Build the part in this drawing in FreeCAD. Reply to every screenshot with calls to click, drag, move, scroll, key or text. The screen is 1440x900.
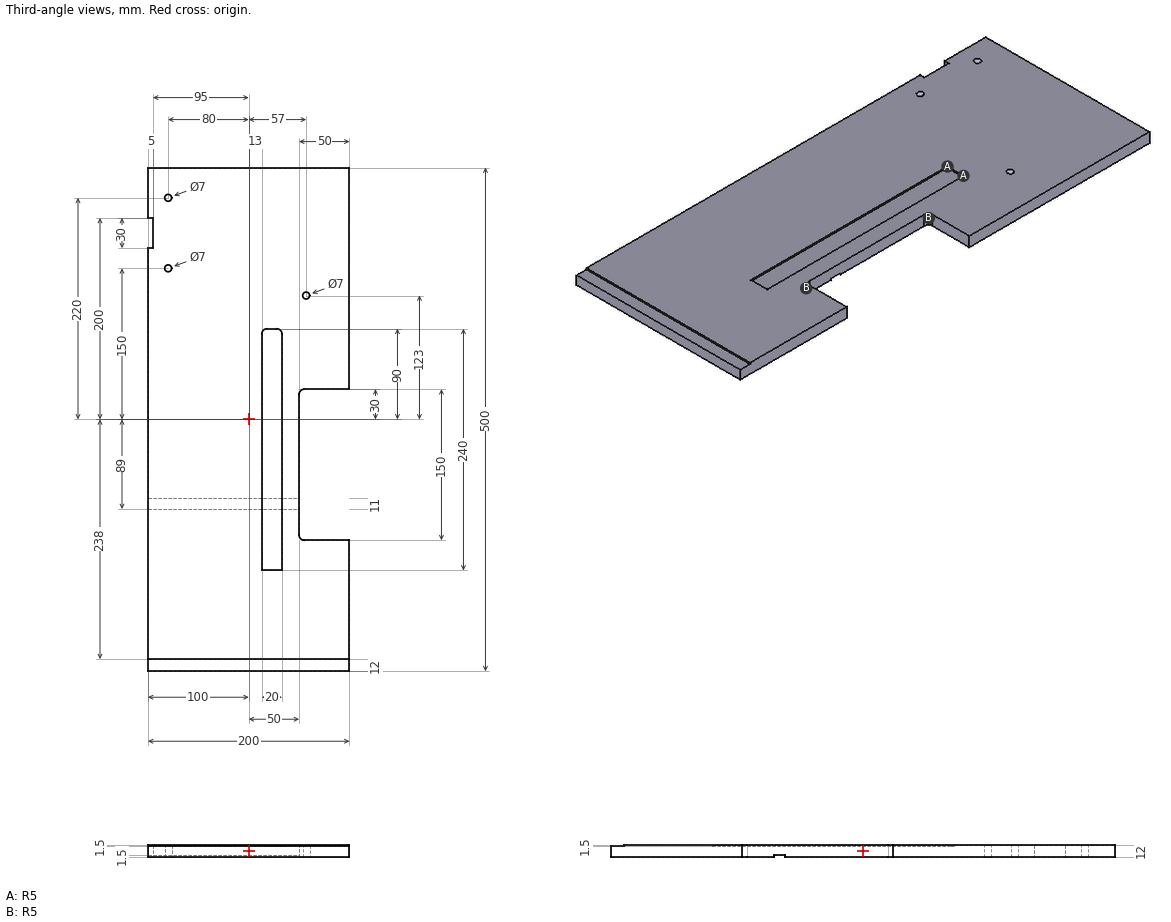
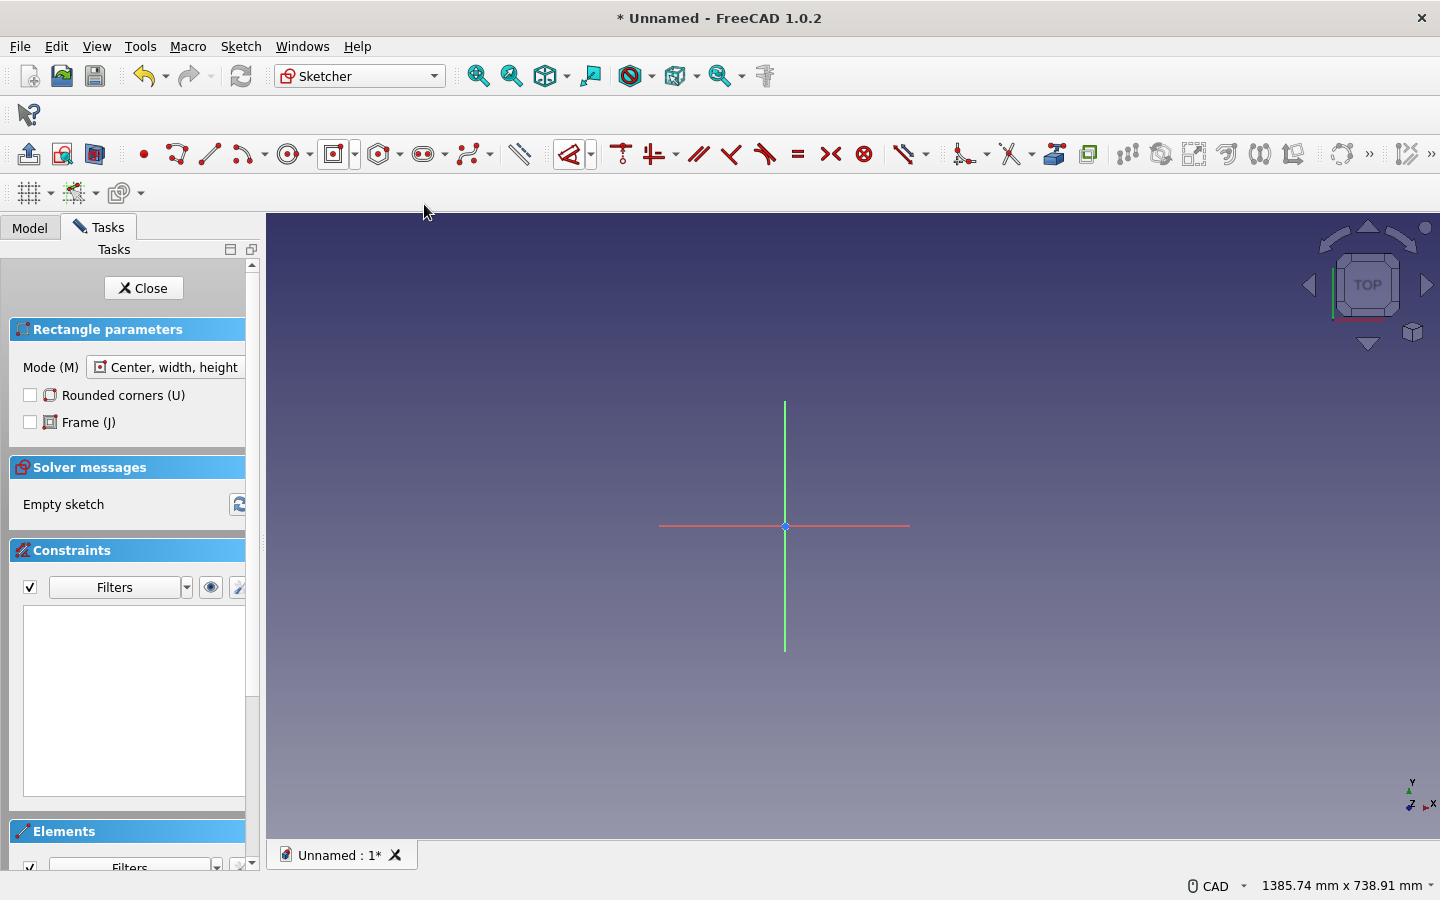
click(785, 526)
move(870, 315)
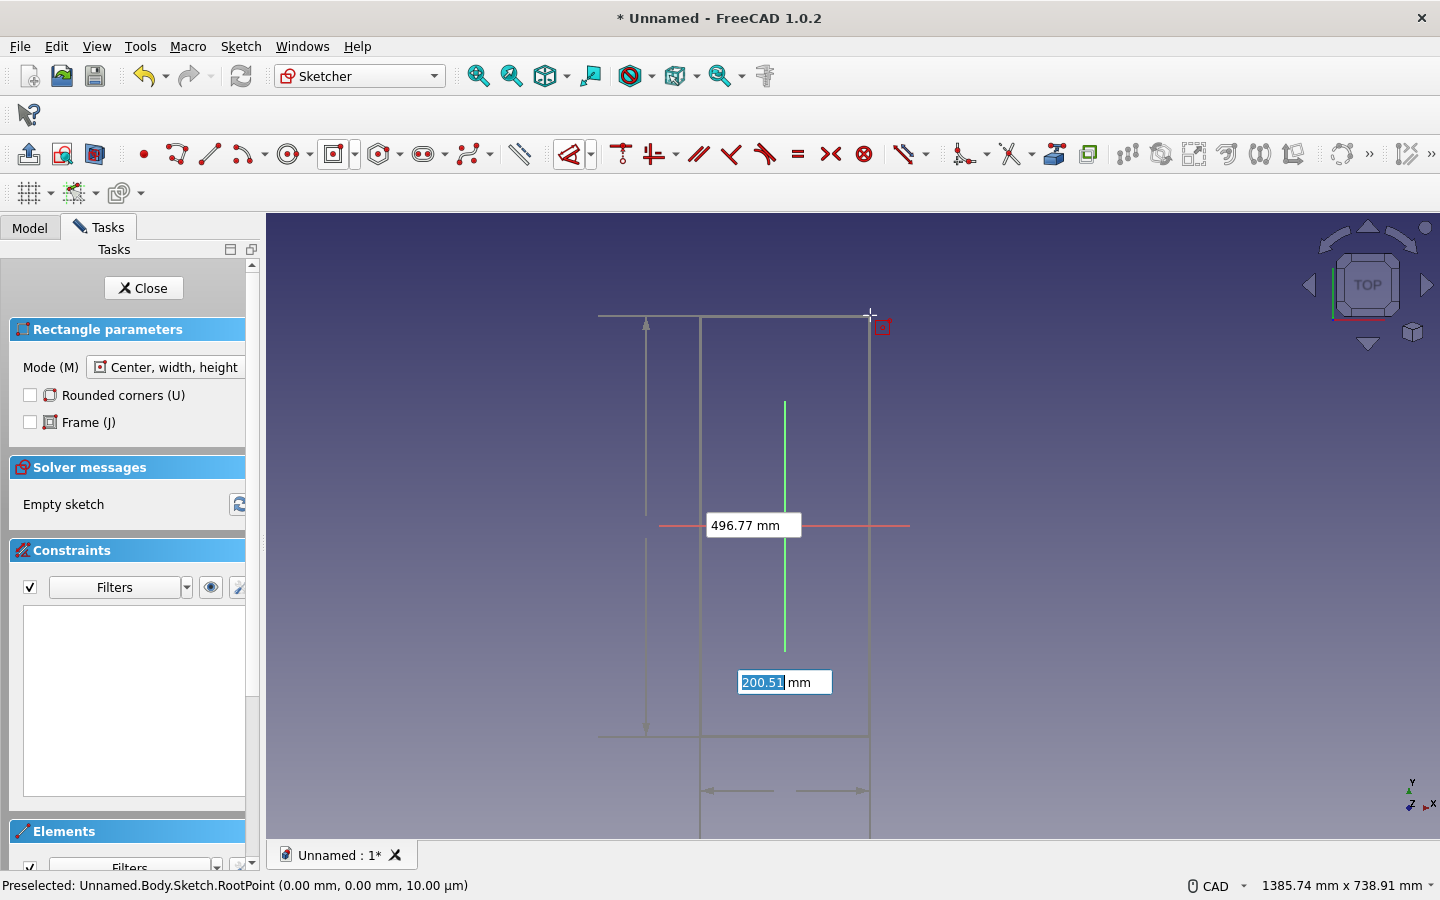
text(200)
key(Tab)
text(500)
key(Return)
key(Escape)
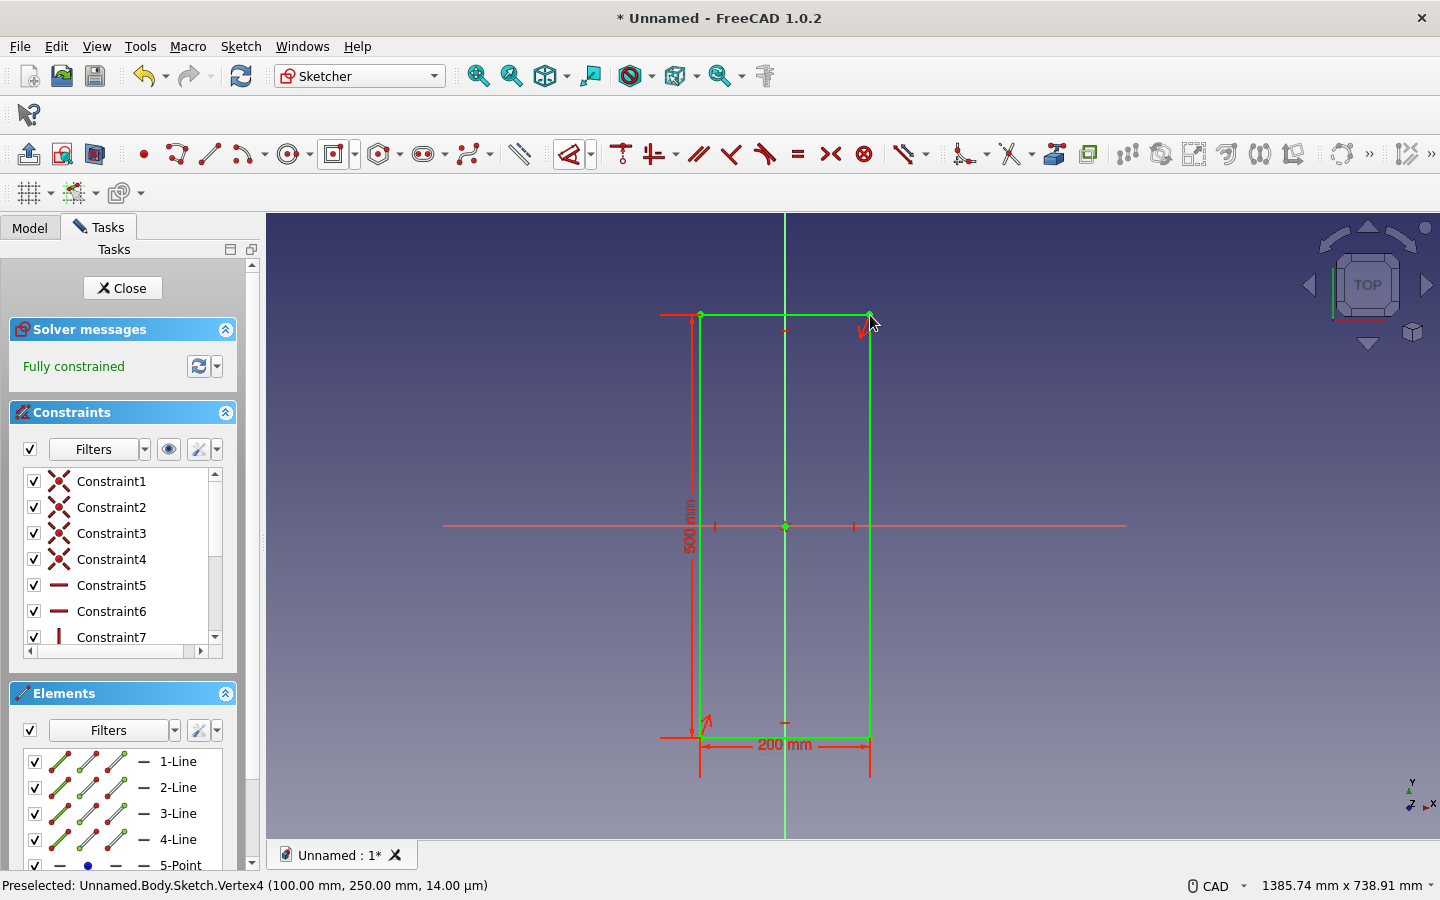
click(123, 288)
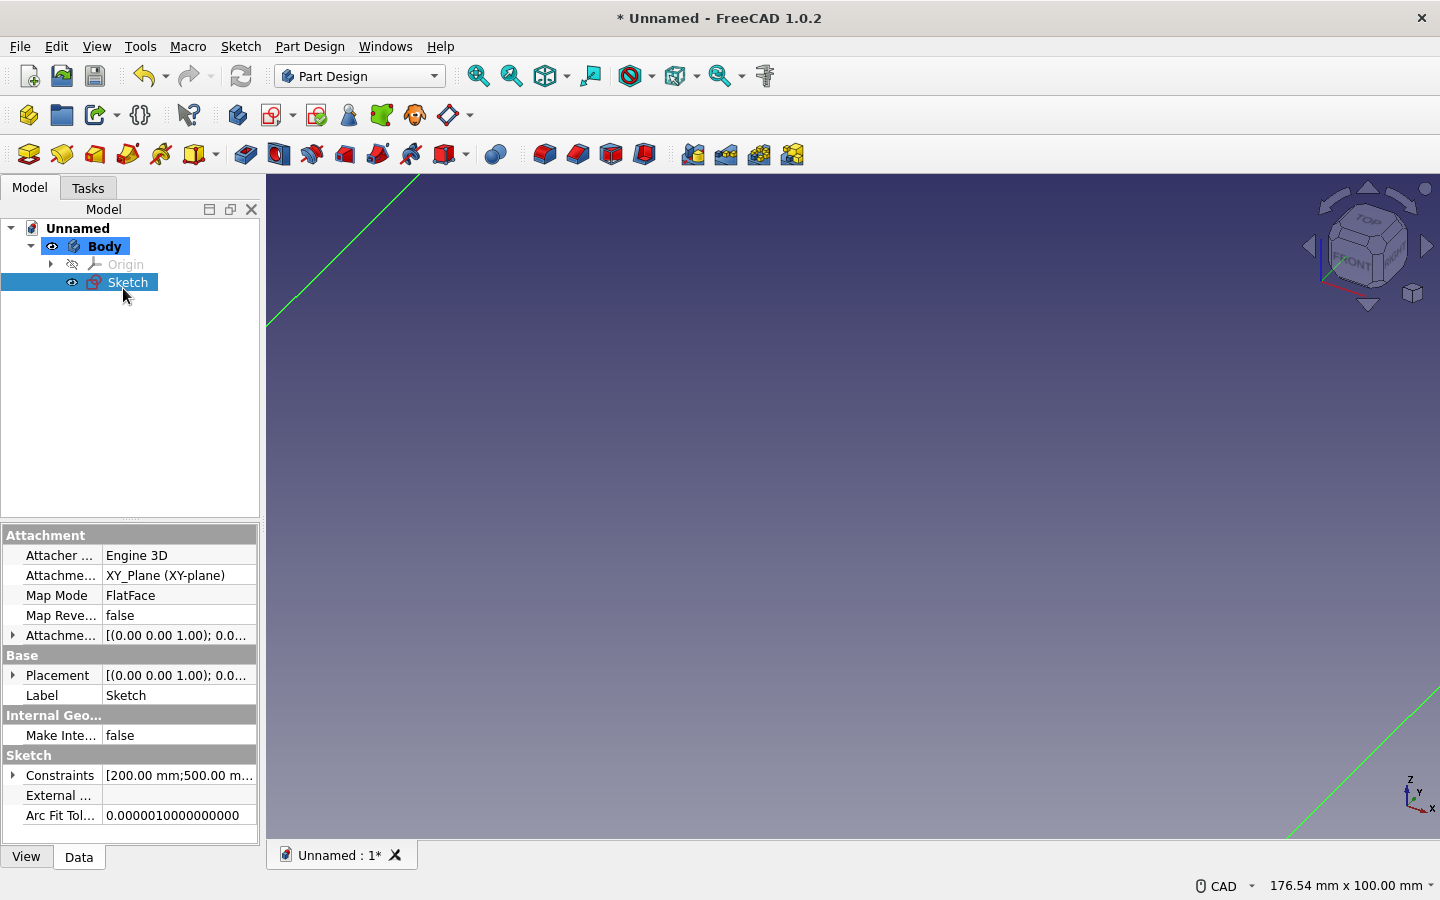
click(29, 154)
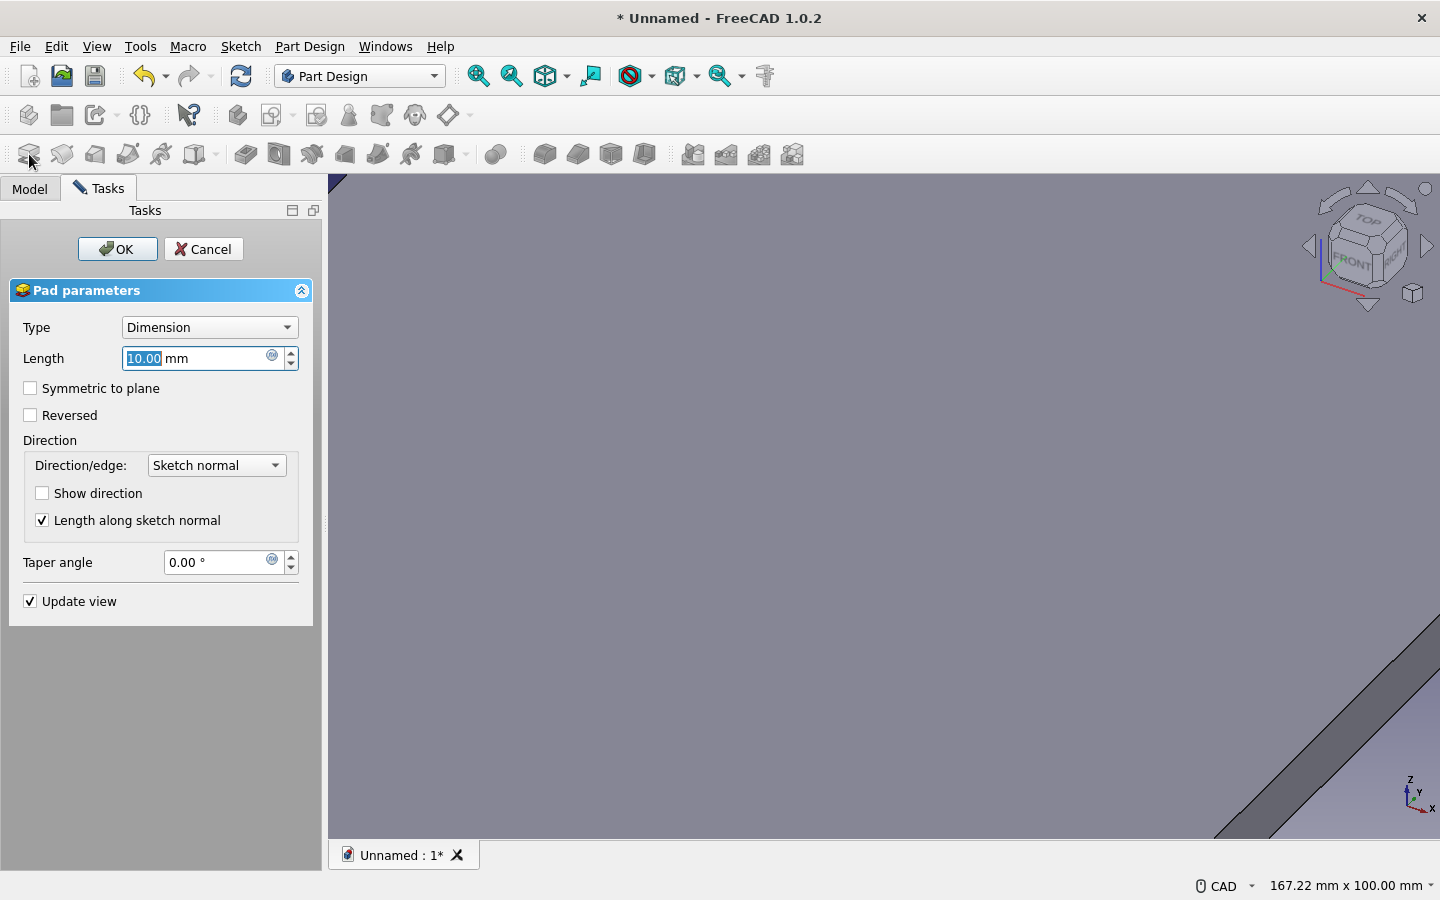
text(12)
key(Tab)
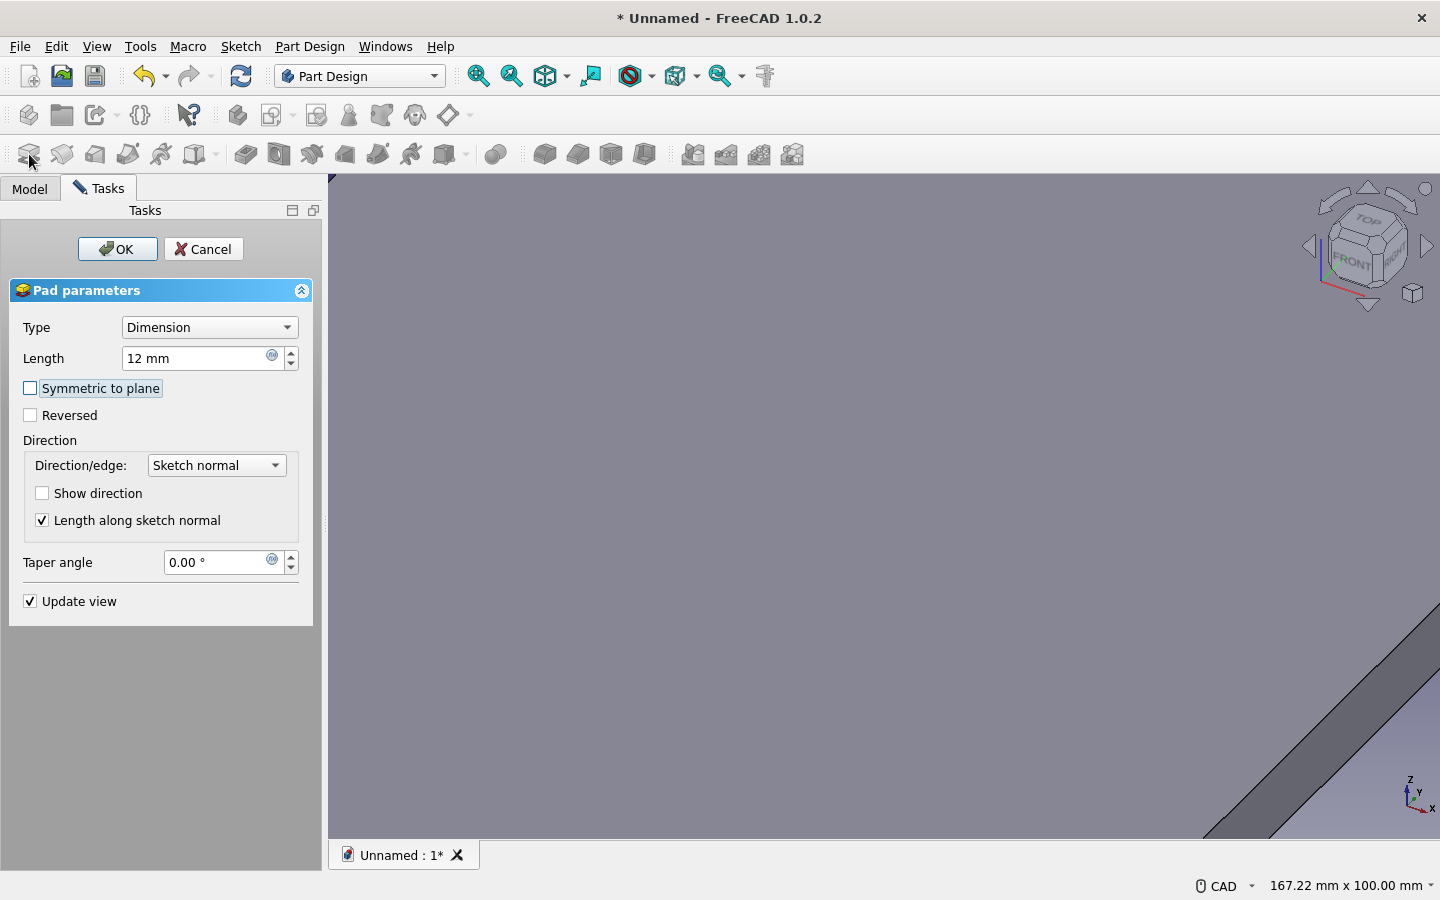
click(31, 388)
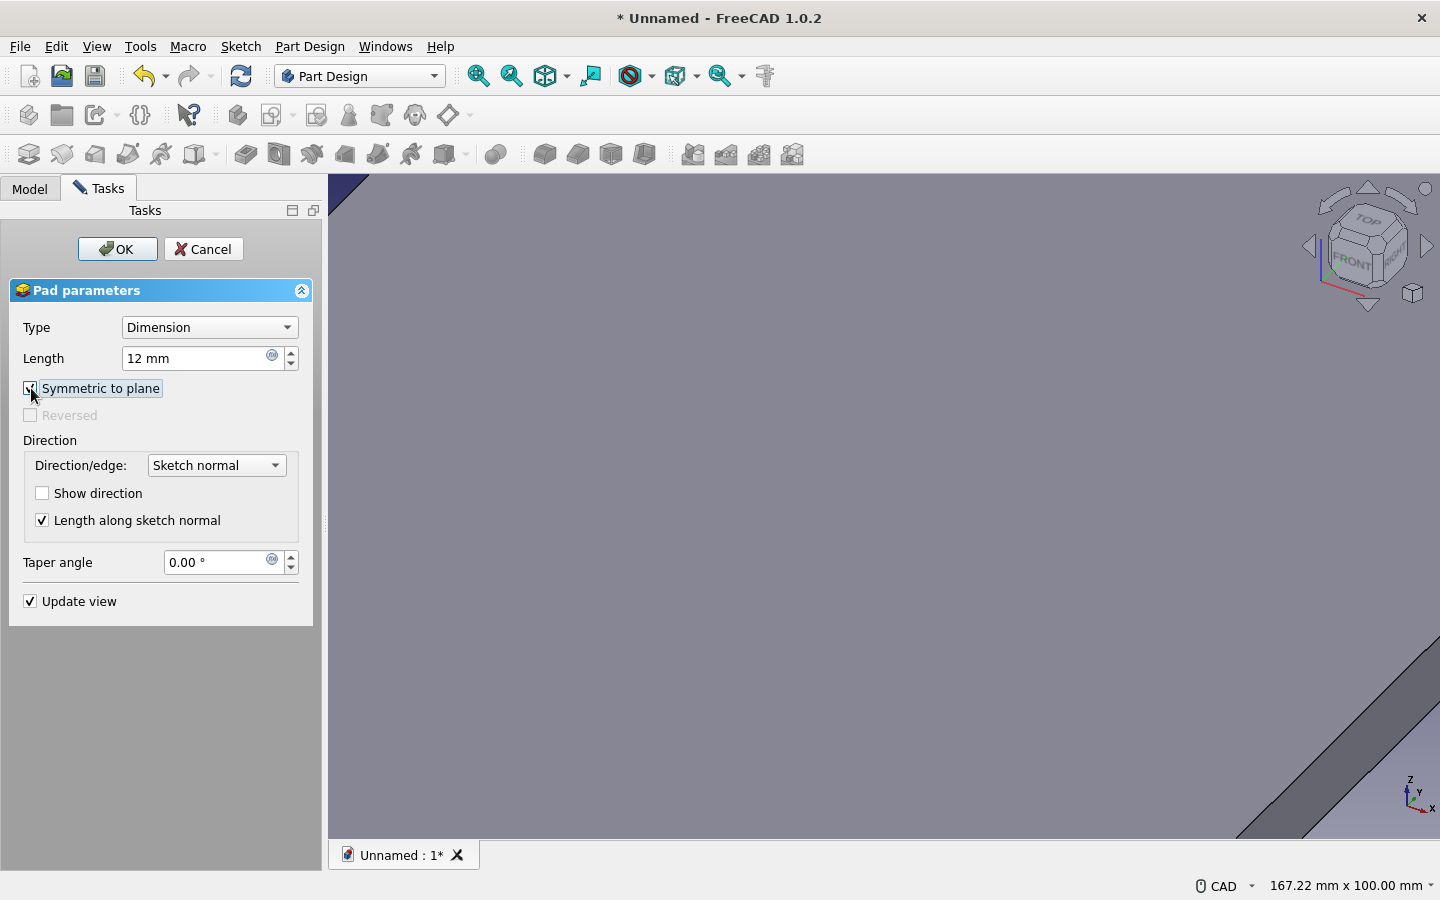
click(118, 249)